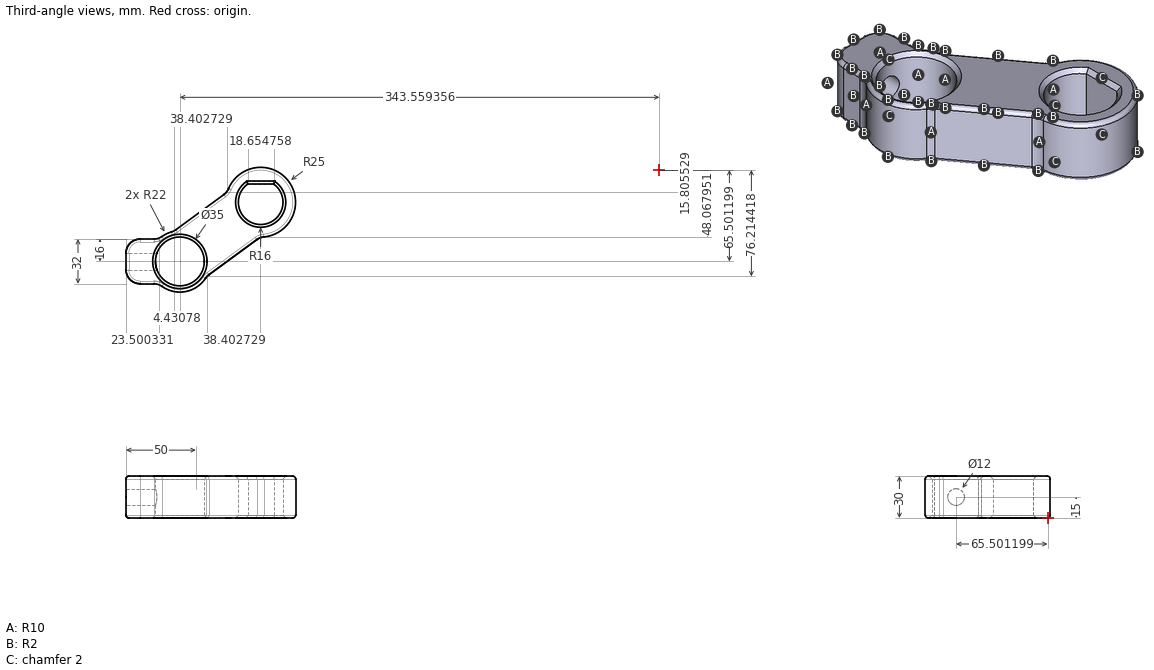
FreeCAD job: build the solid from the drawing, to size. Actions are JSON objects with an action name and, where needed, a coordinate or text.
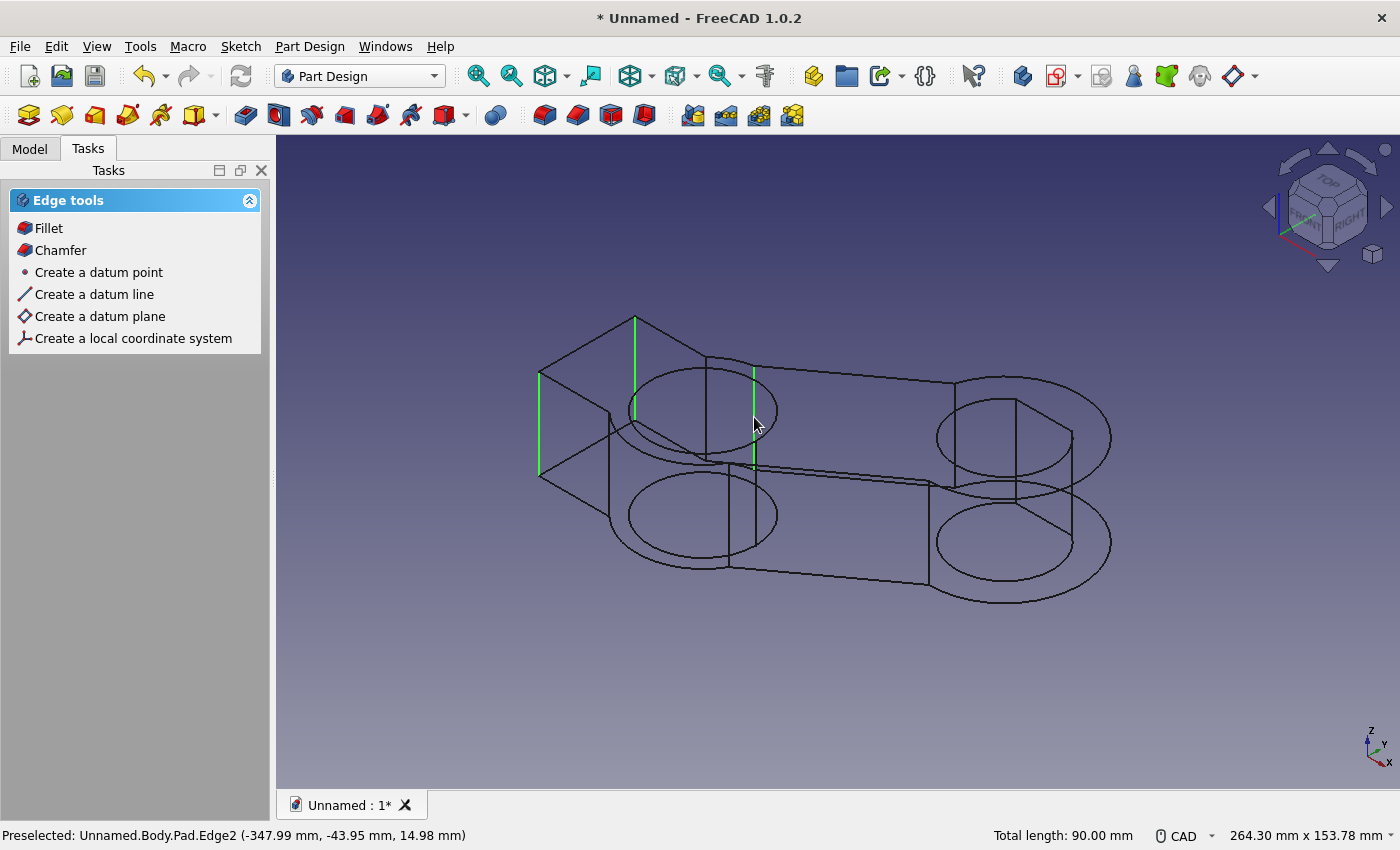
{"action": "left_click", "coordinate": [955, 435], "text": "ctrl"}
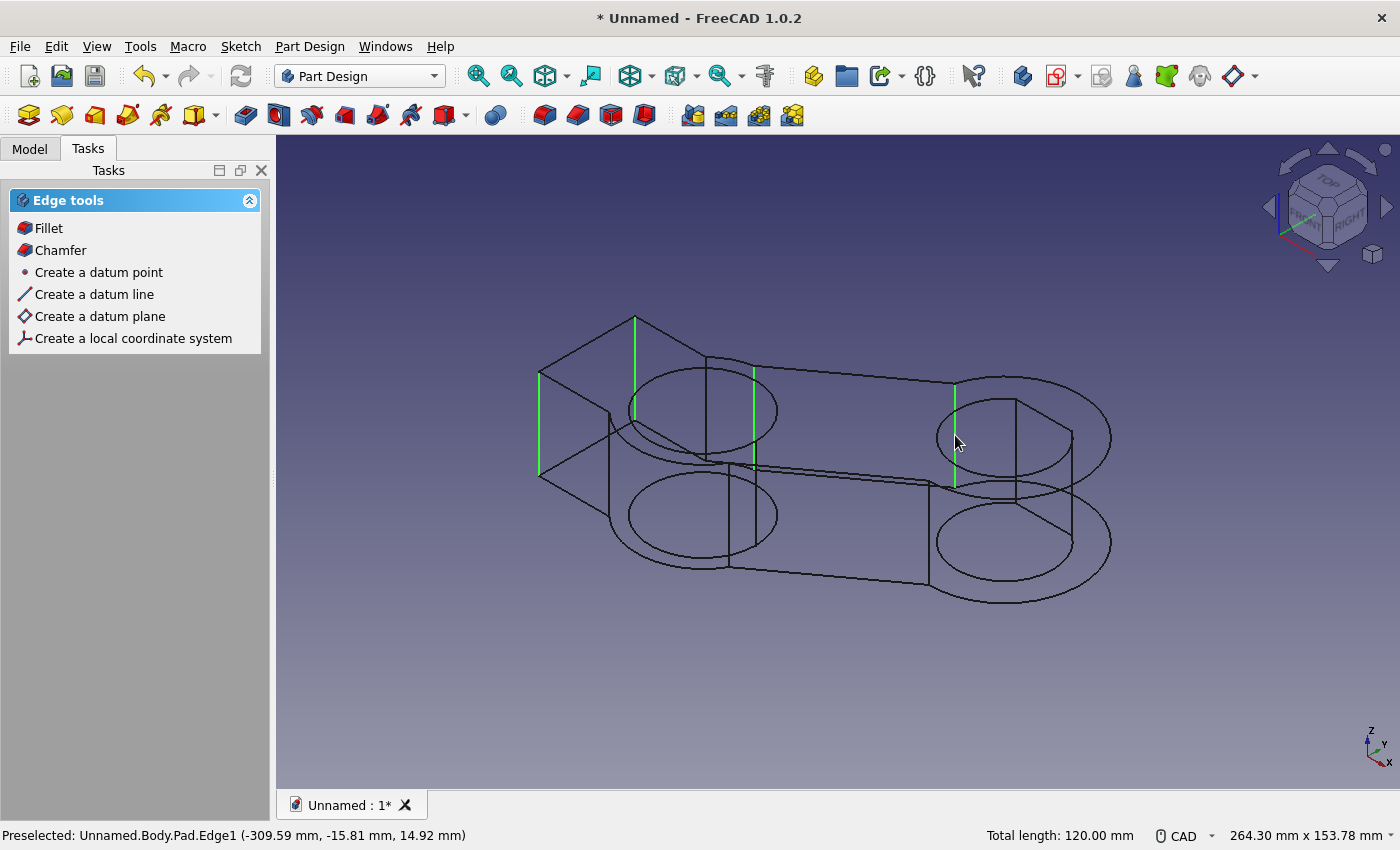
{"action": "left_click", "coordinate": [929, 532], "text": "ctrl"}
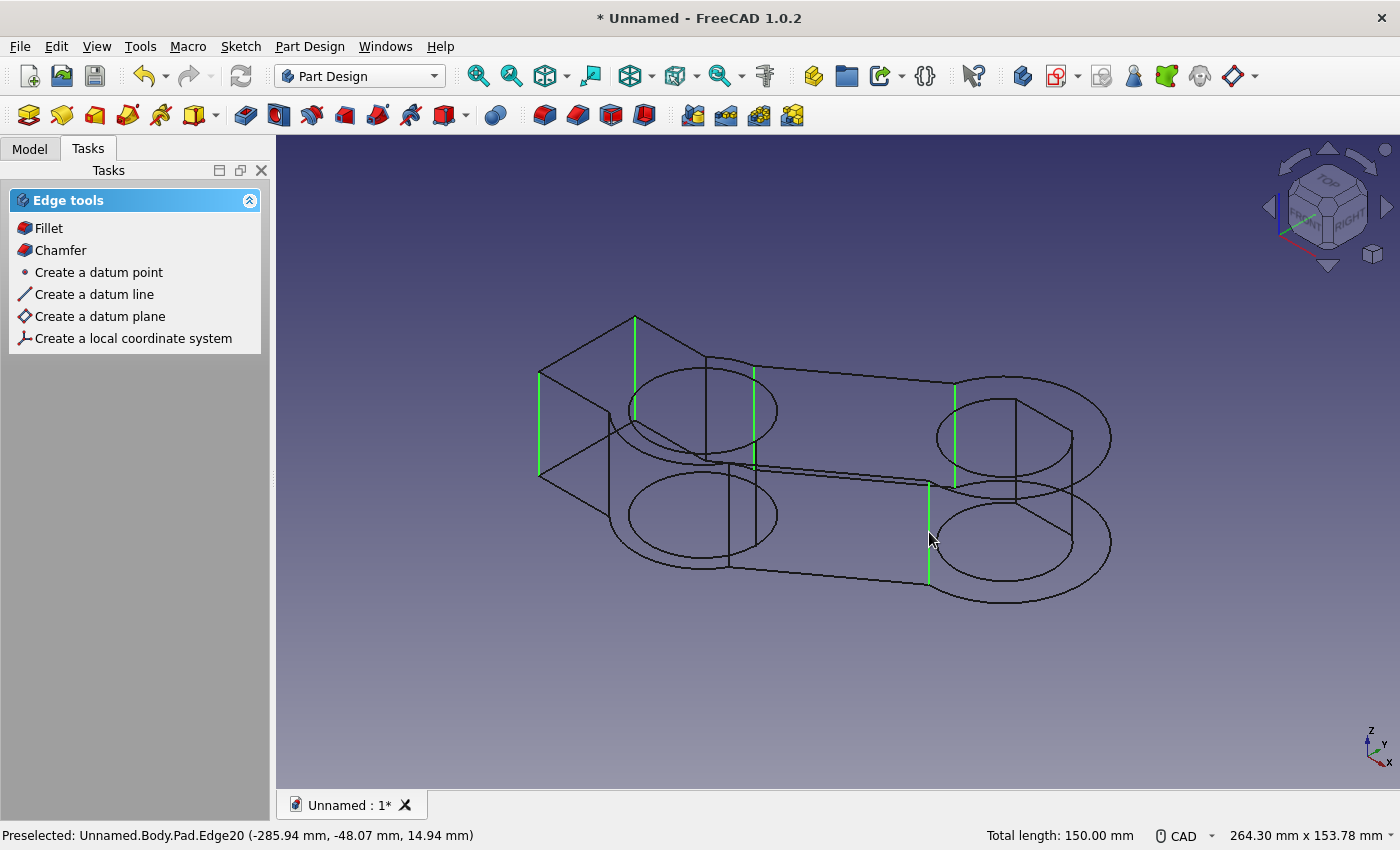
{"action": "left_click", "coordinate": [729, 514], "text": "ctrl"}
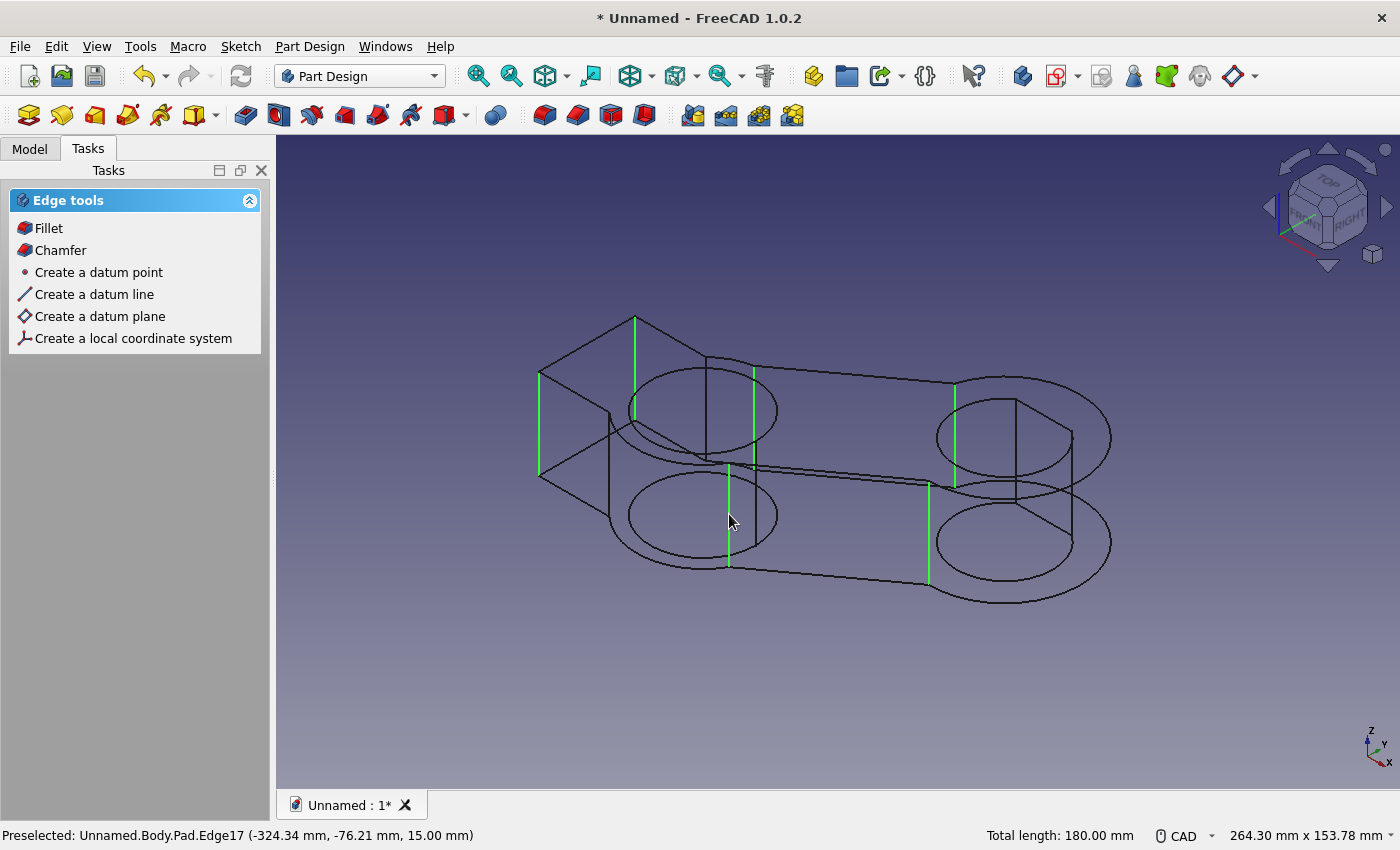
{"action": "left_click", "coordinate": [609, 464], "text": "ctrl"}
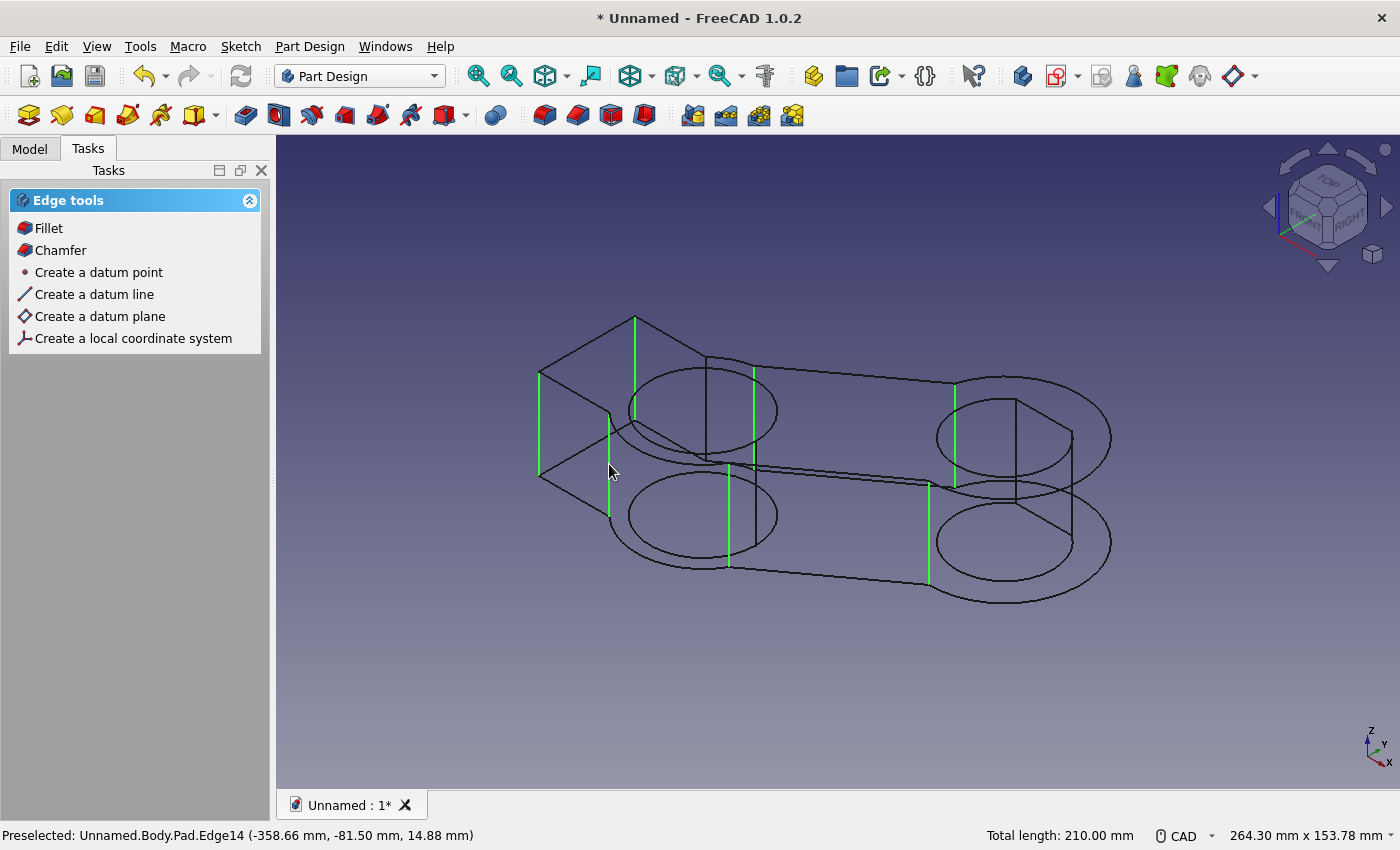
{"action": "left_click", "coordinate": [706, 408], "text": "ctrl"}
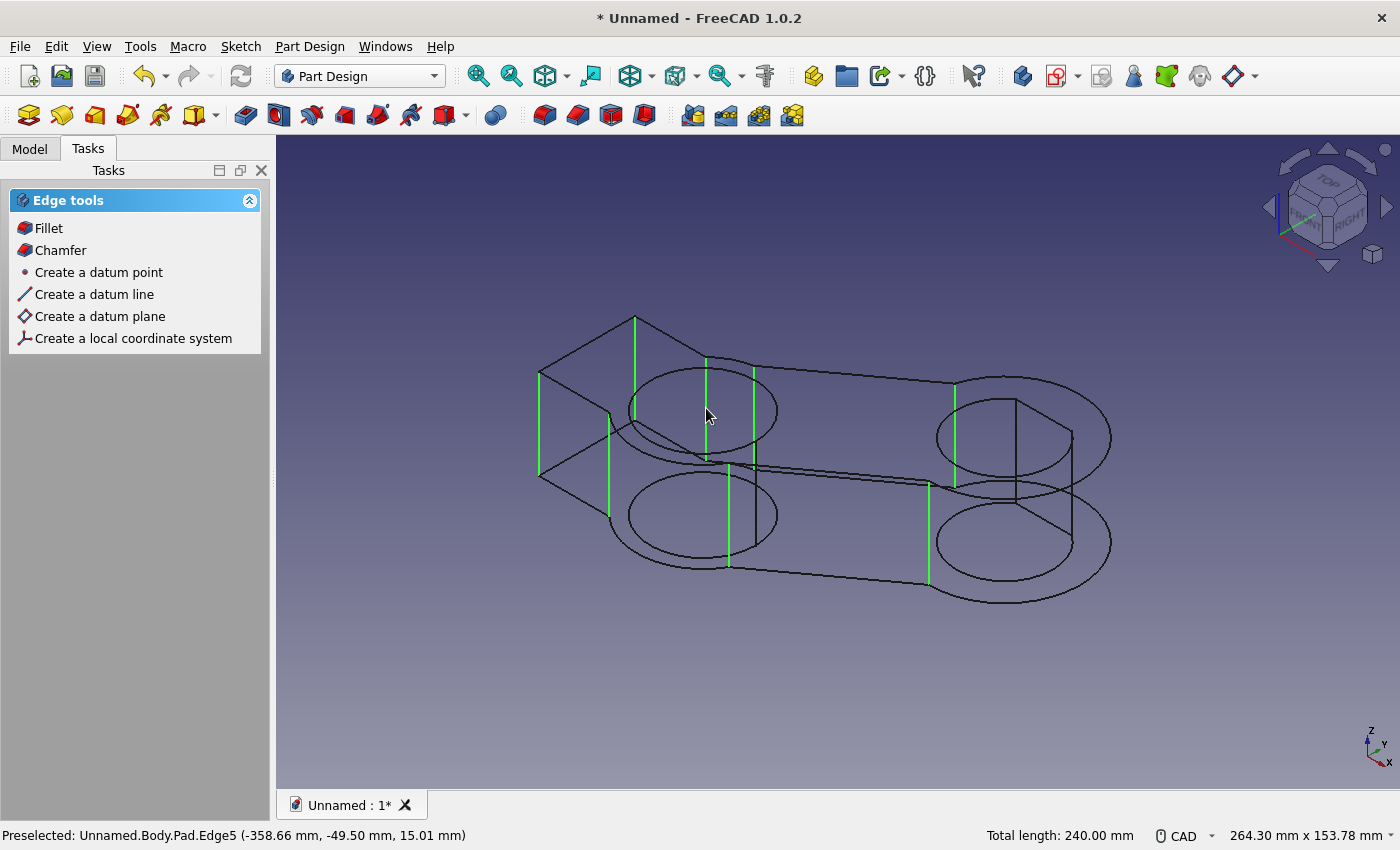
{"action": "key", "text": "v 1"}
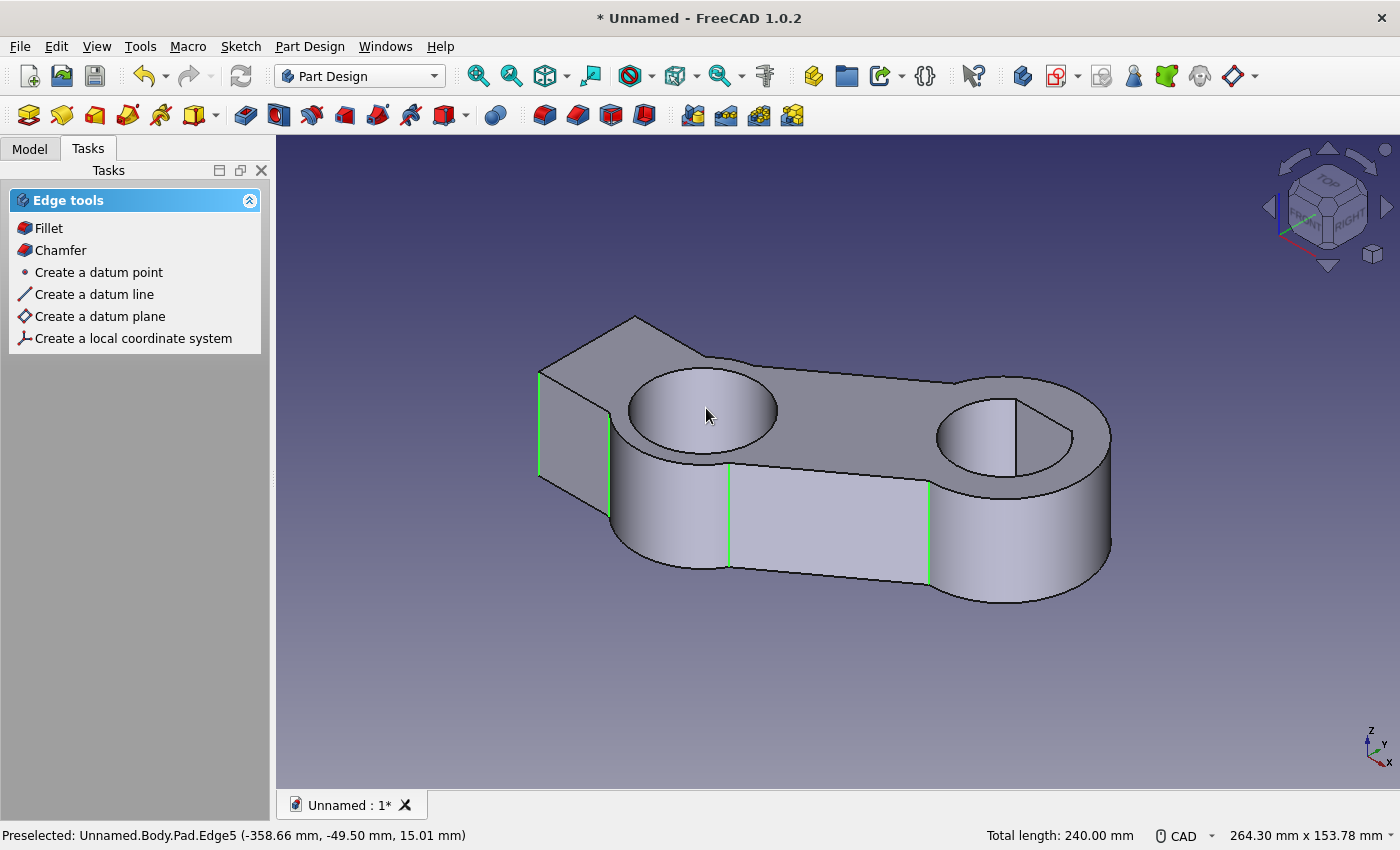
{"action": "left_click", "coordinate": [545, 116]}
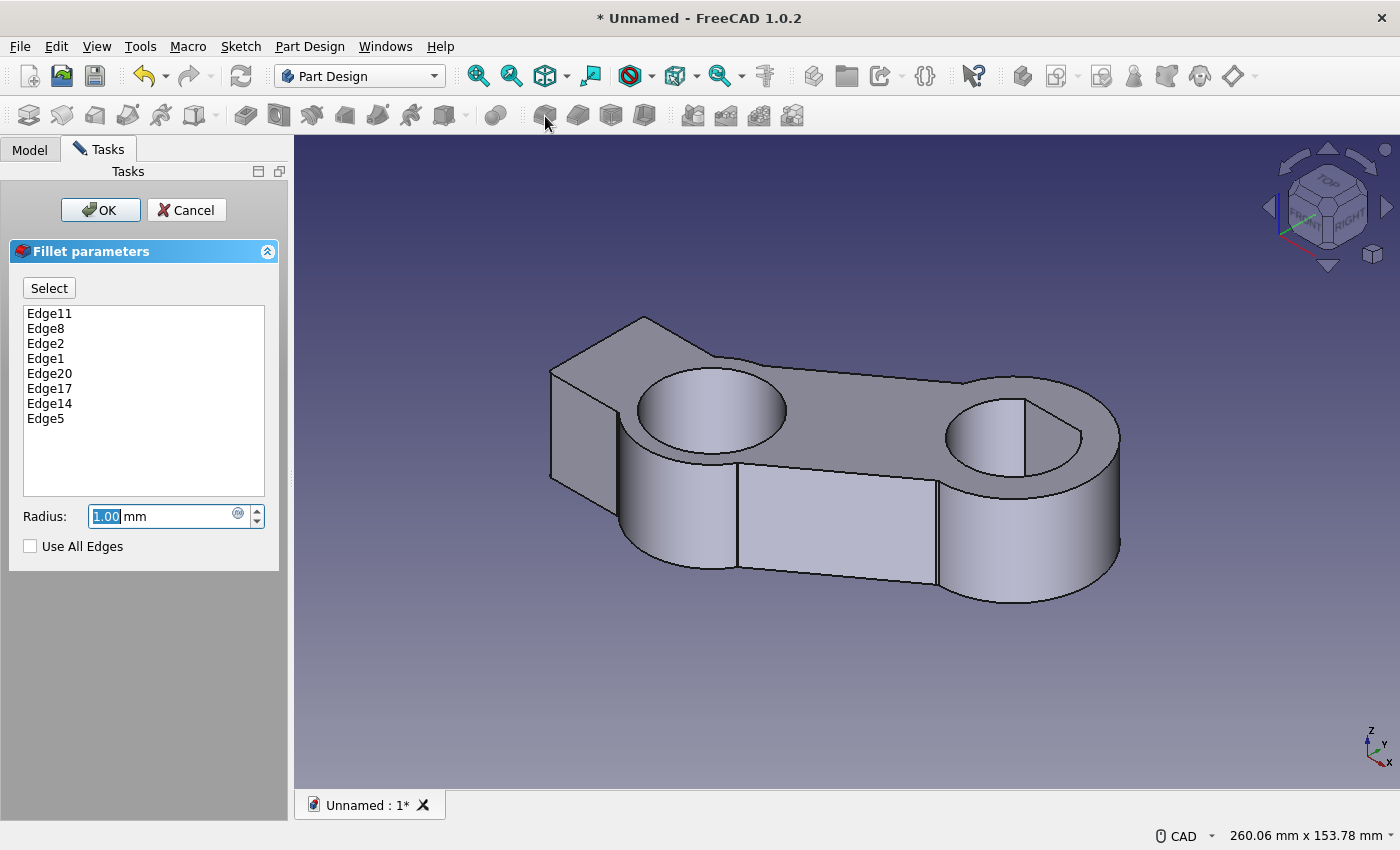
{"action": "type", "text": "10"}
{"action": "key", "text": "Tab"}